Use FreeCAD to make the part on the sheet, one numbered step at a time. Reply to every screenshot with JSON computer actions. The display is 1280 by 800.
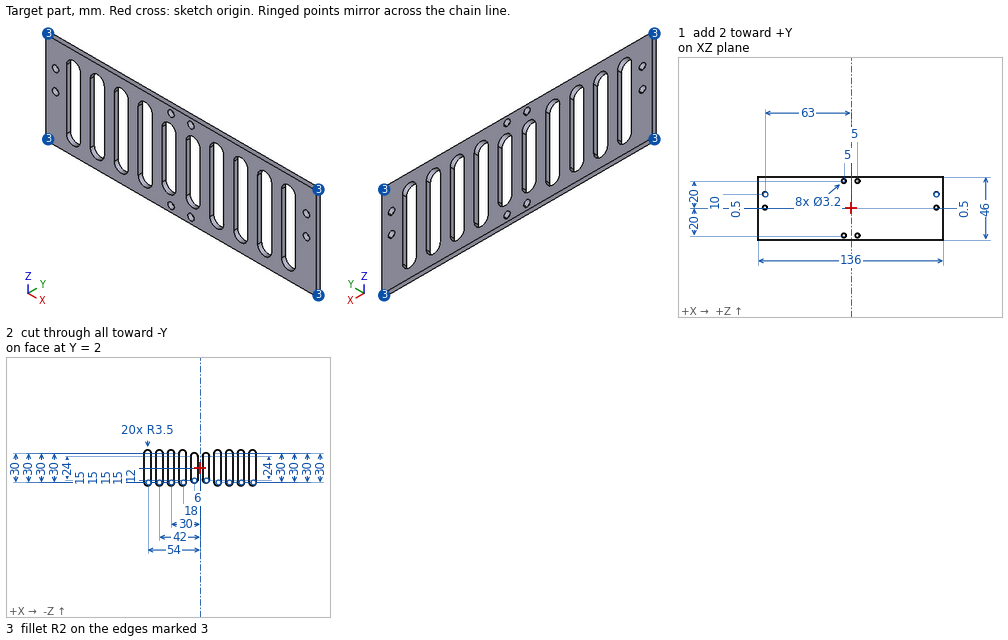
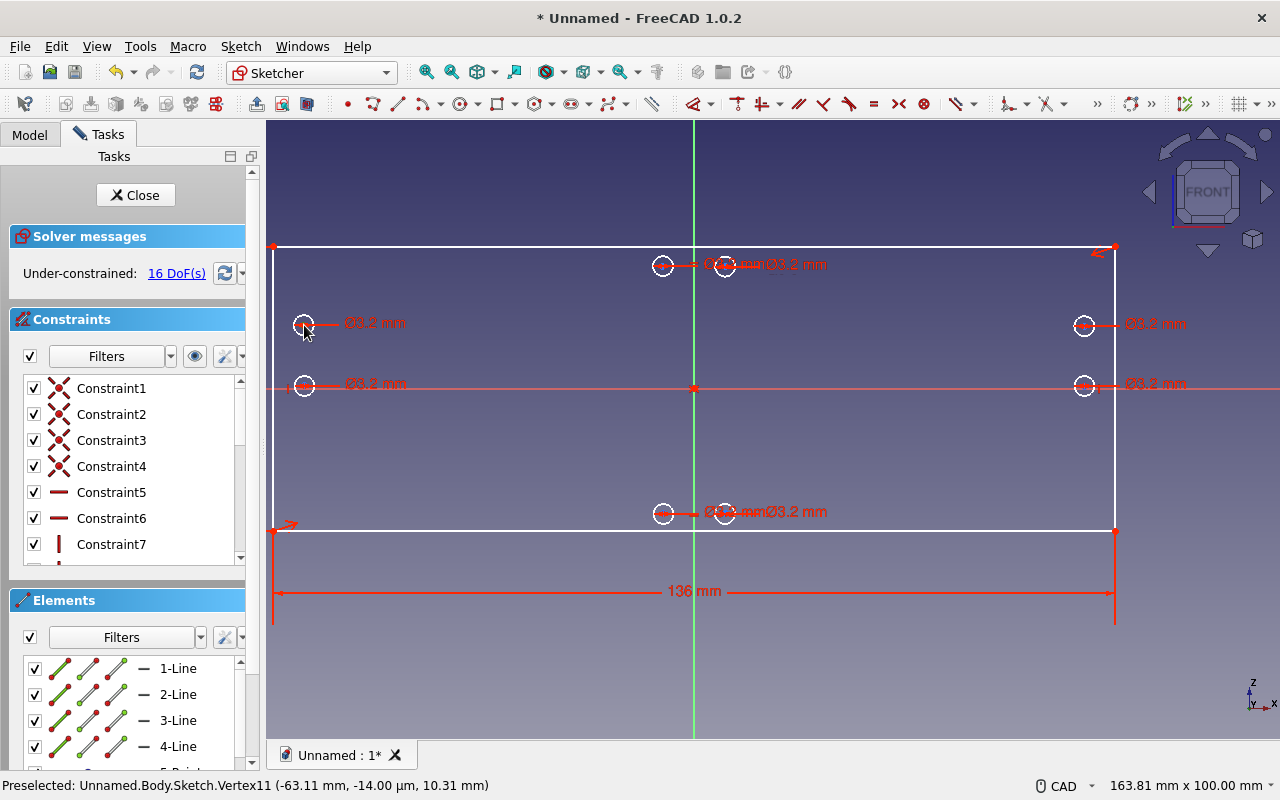
{"action": "left_click", "coordinate": [304, 386]}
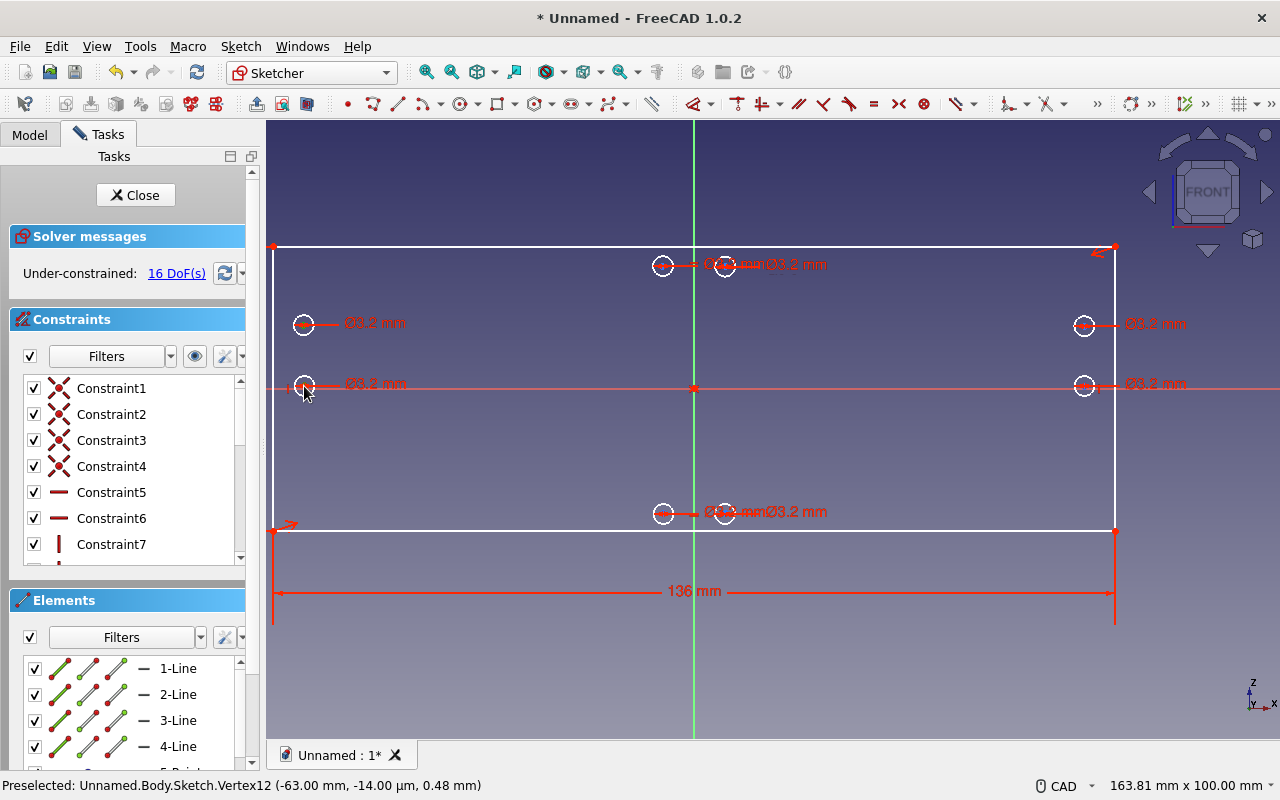
{"action": "key", "text": "v"}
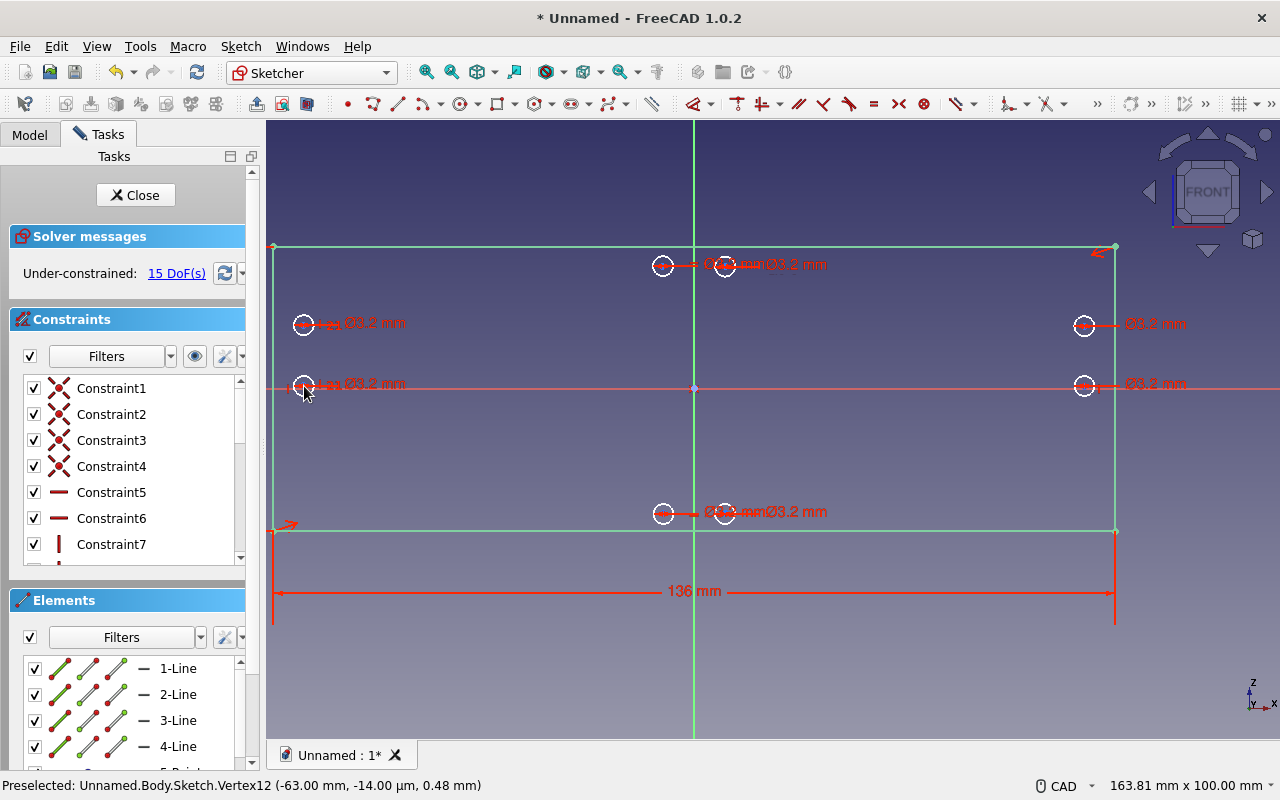
{"action": "left_click", "coordinate": [663, 266]}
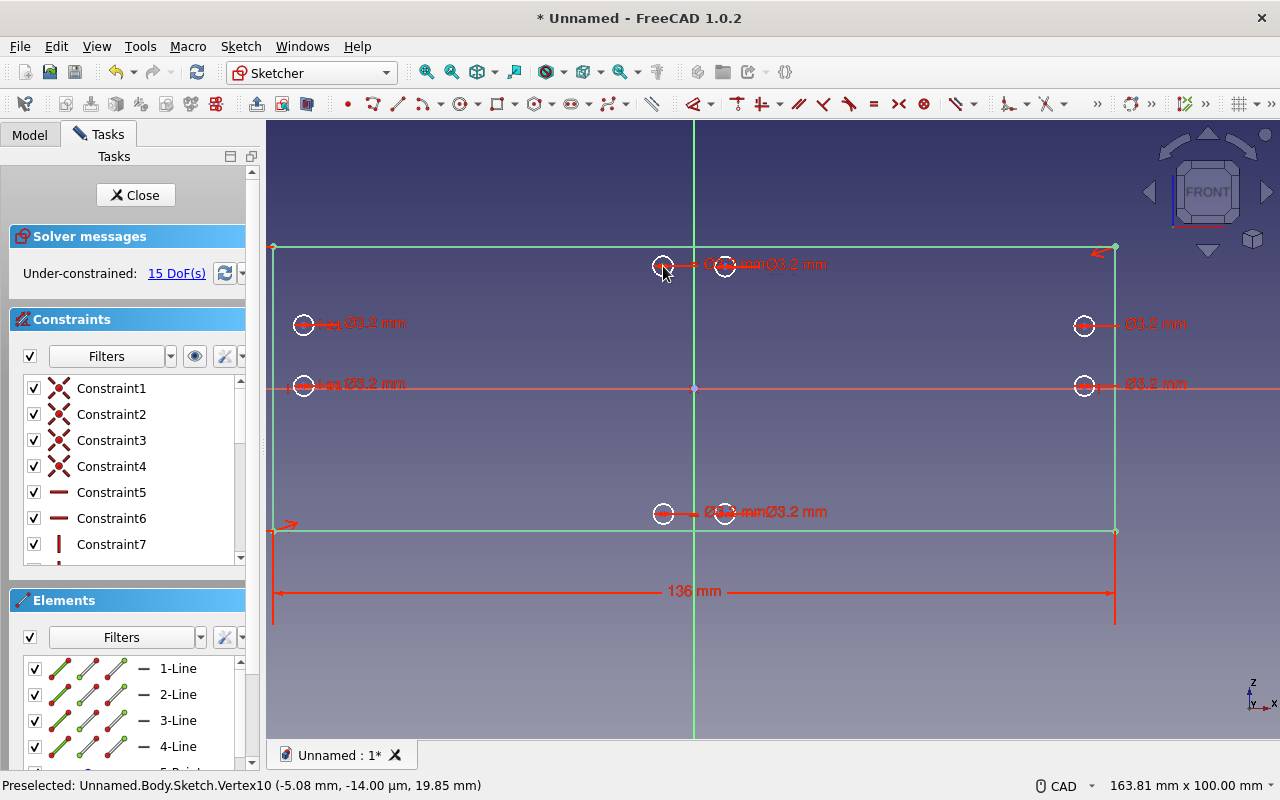
{"action": "left_click", "coordinate": [725, 267]}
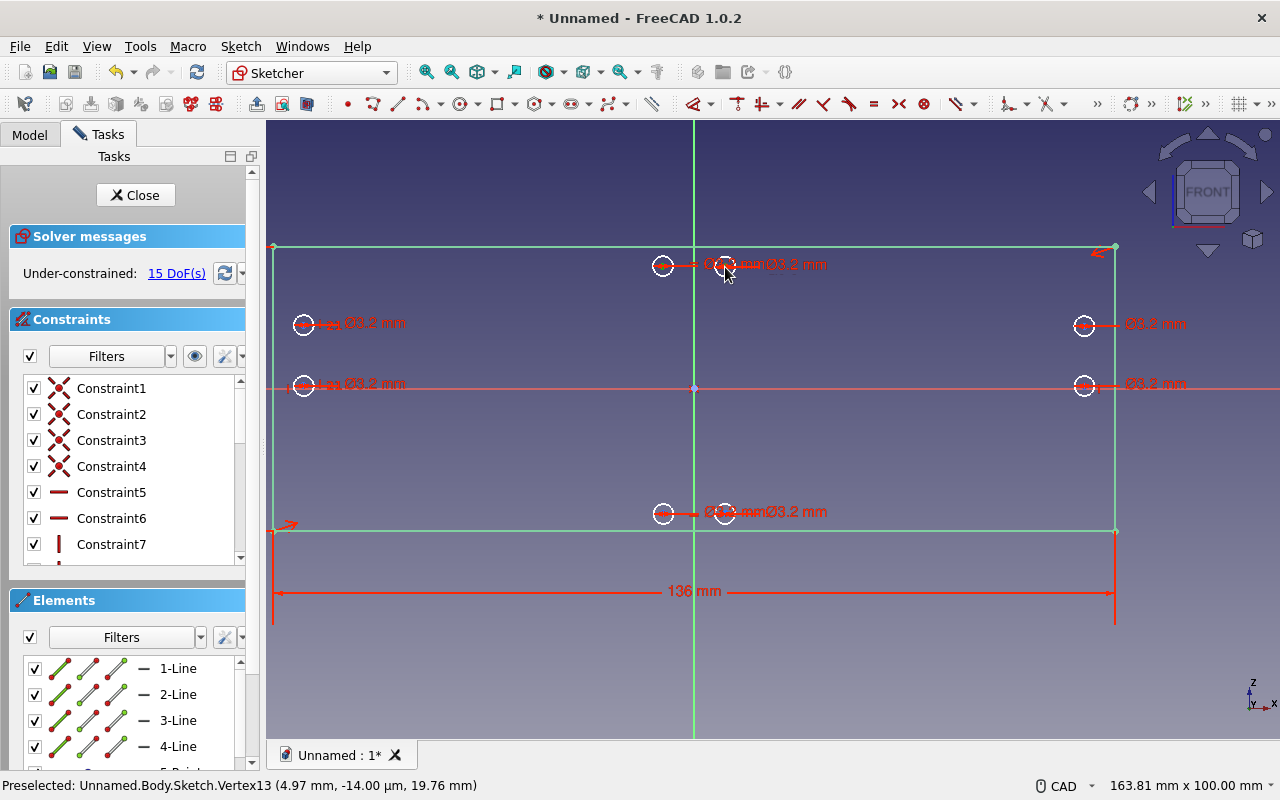
{"action": "left_click", "coordinate": [780, 104]}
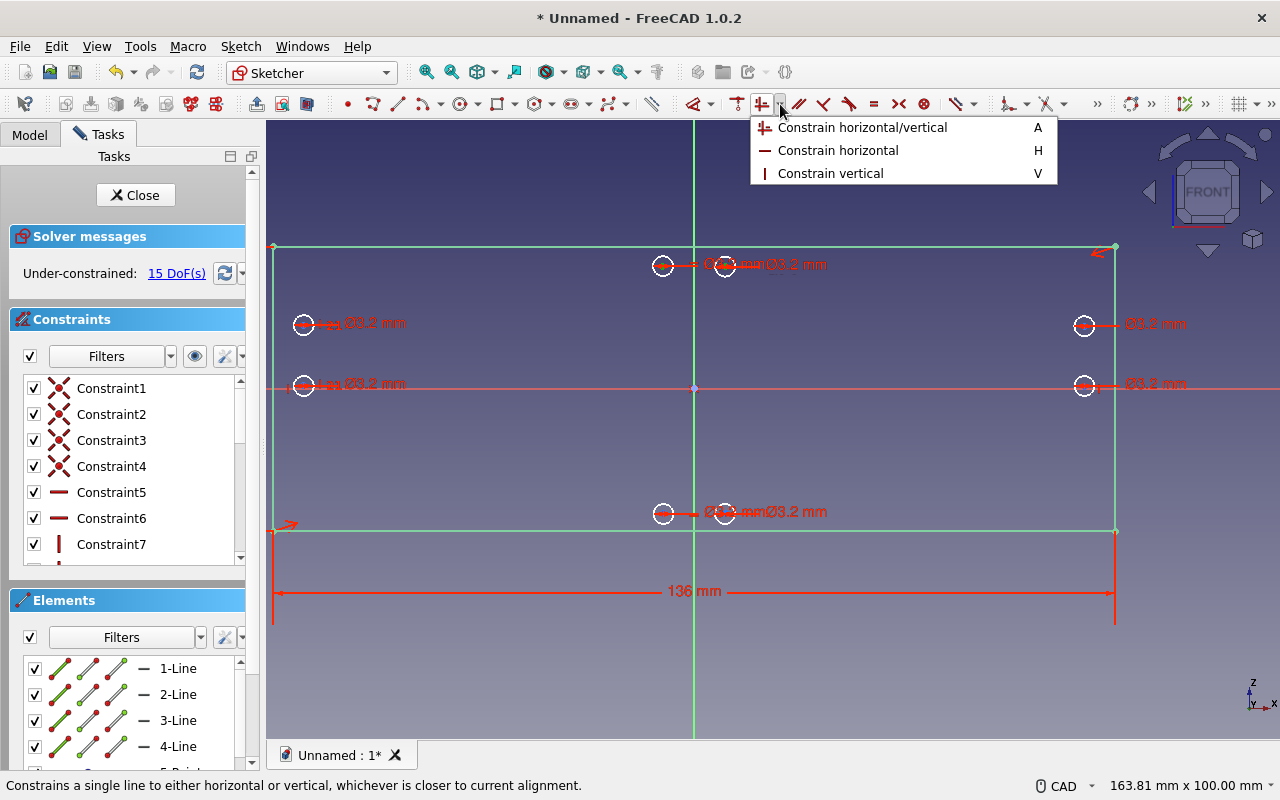
{"action": "left_click", "coordinate": [904, 150]}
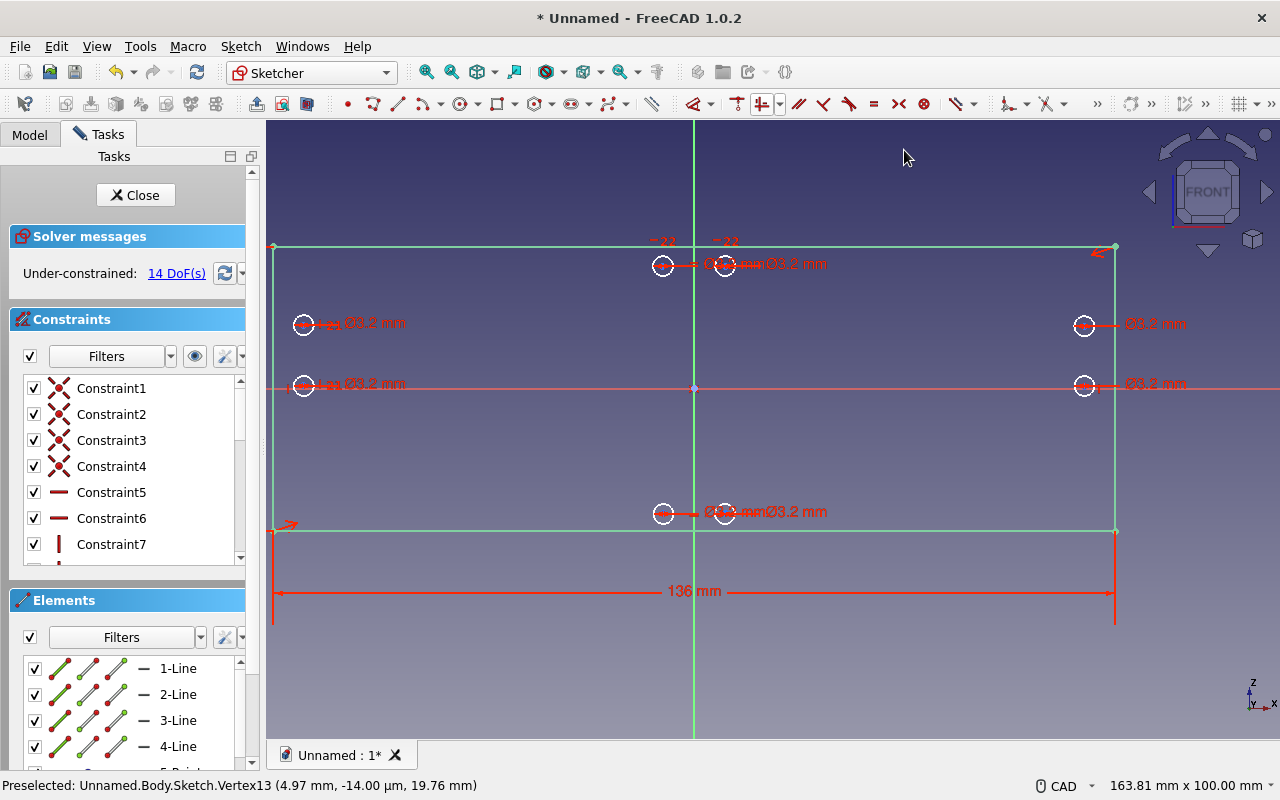
{"action": "left_click", "coordinate": [1084, 326]}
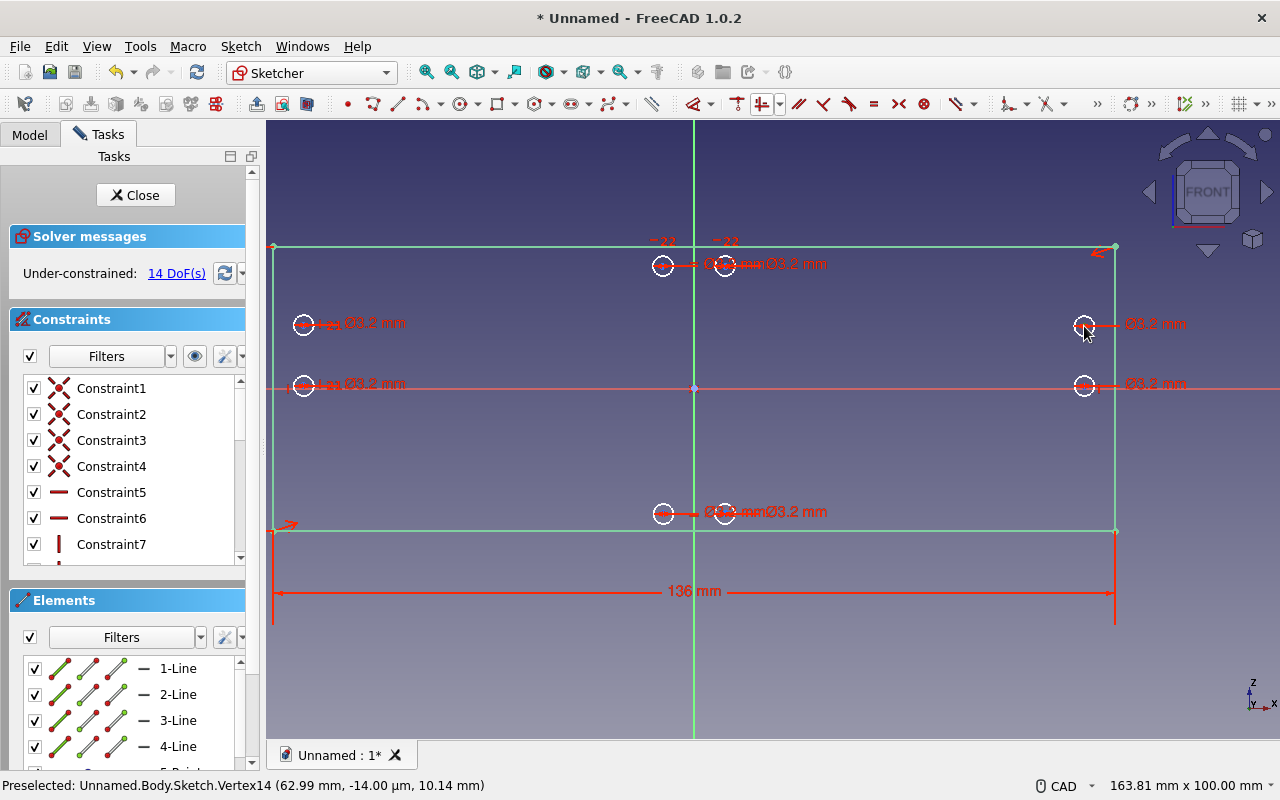
{"action": "left_click", "coordinate": [1084, 386]}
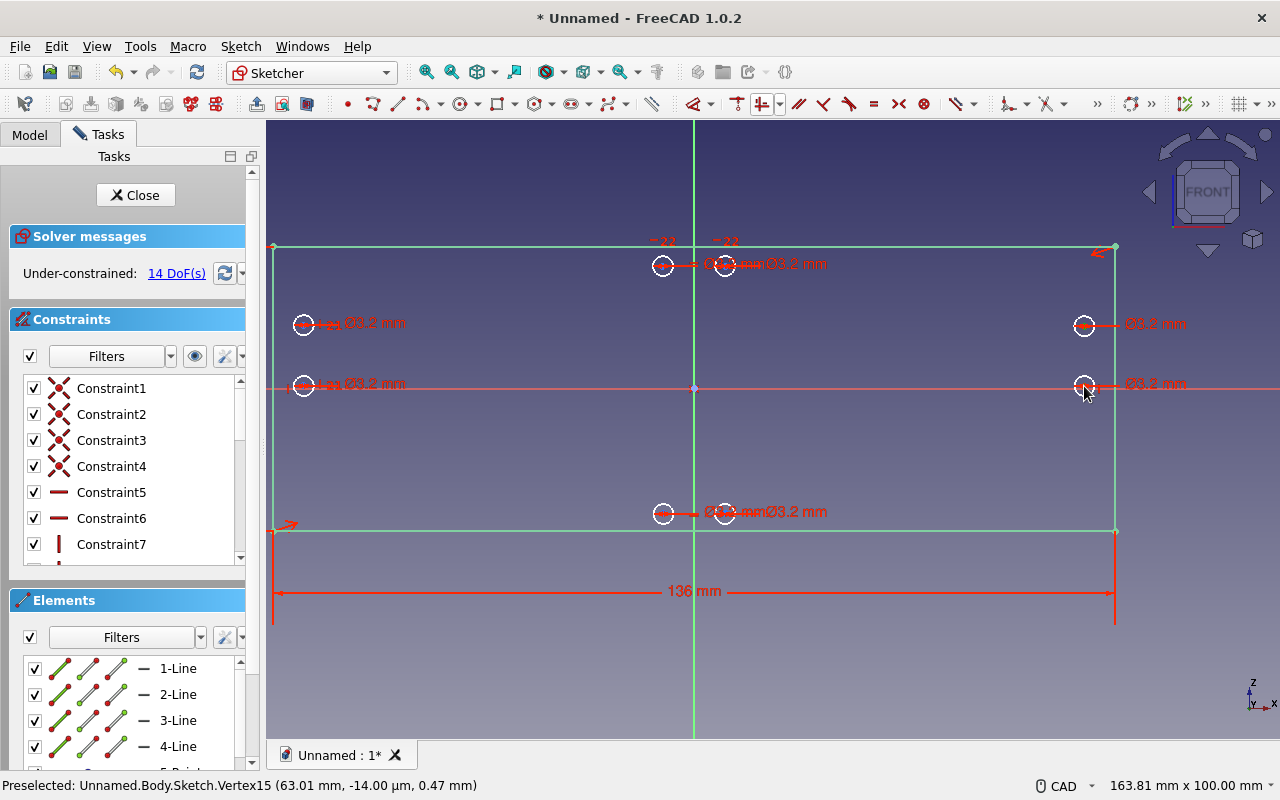
{"action": "key", "text": "v"}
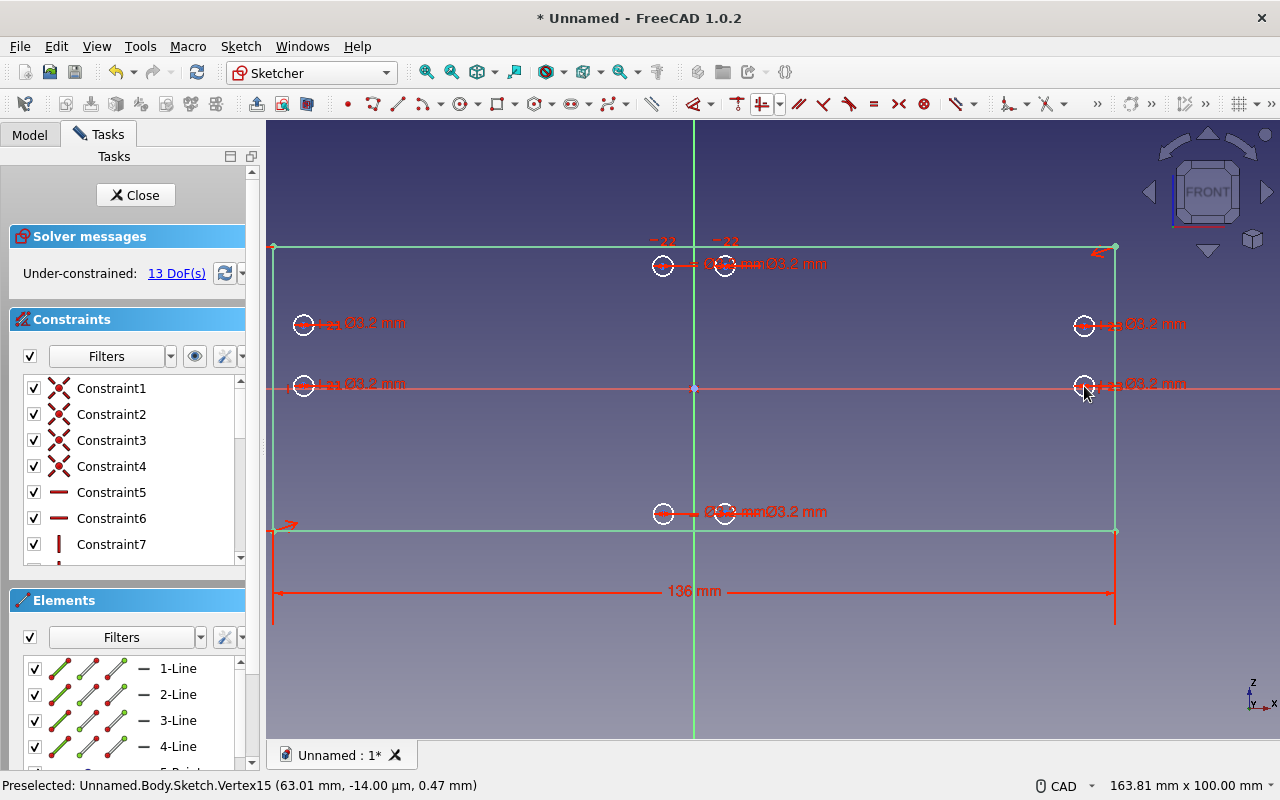
{"action": "left_click", "coordinate": [663, 266]}